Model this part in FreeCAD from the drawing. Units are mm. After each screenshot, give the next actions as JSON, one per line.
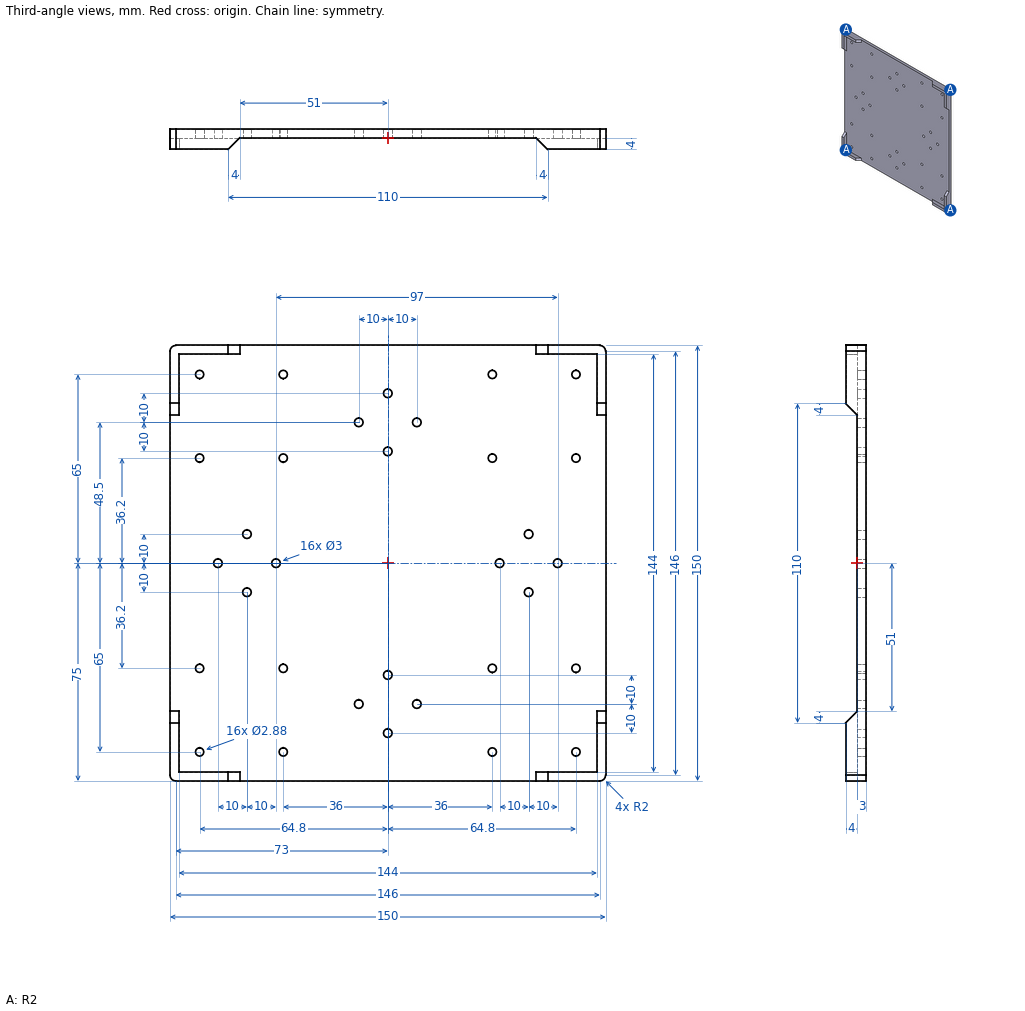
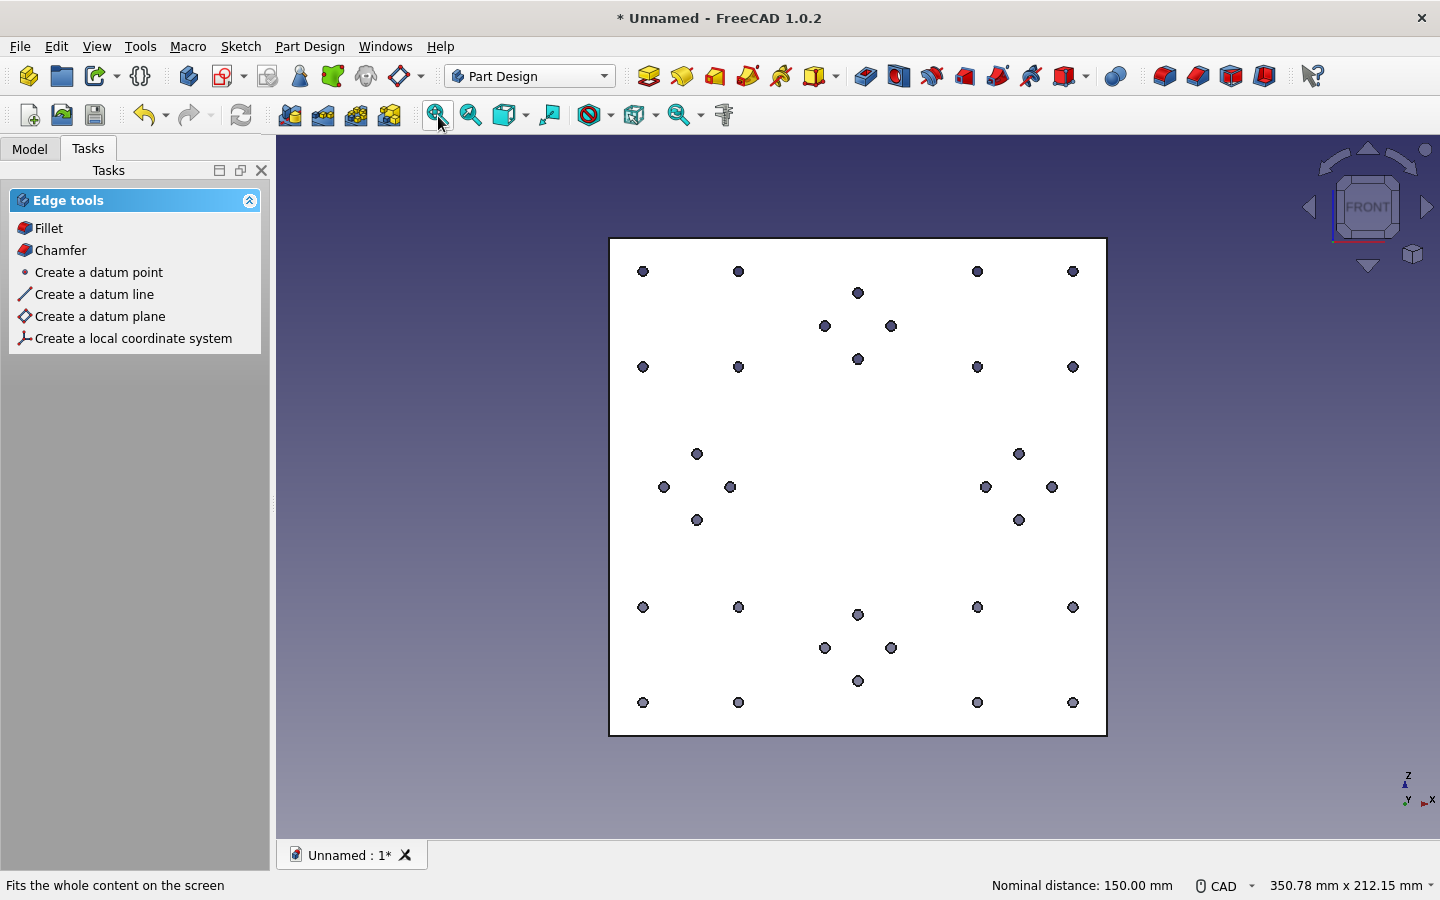
{"action": "key", "text": "3"}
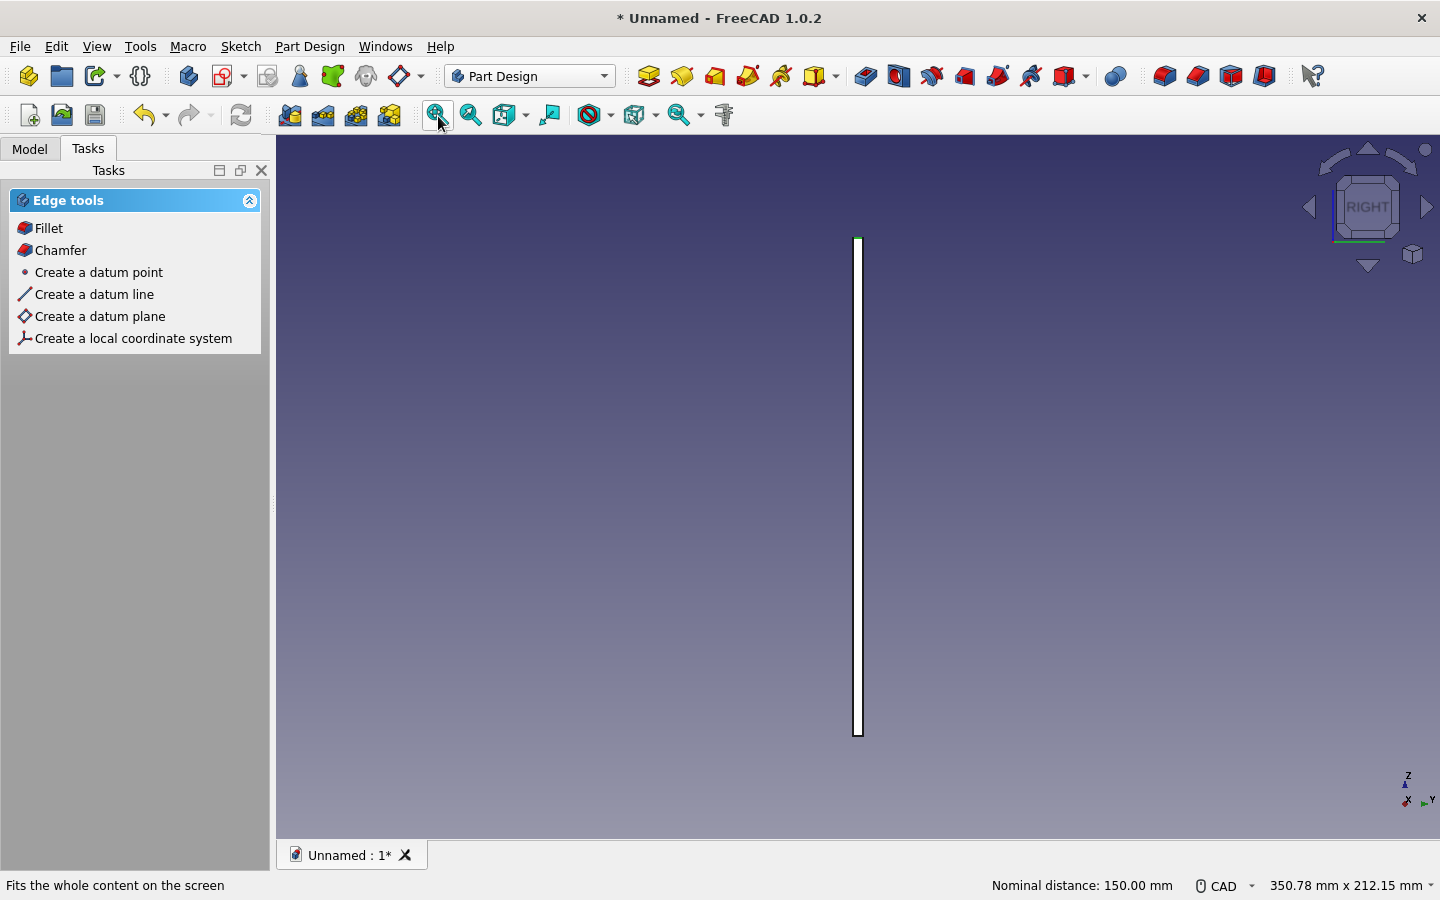
{"action": "scroll", "coordinate": [858, 735], "scroll_direction": "up", "scroll_amount": 7}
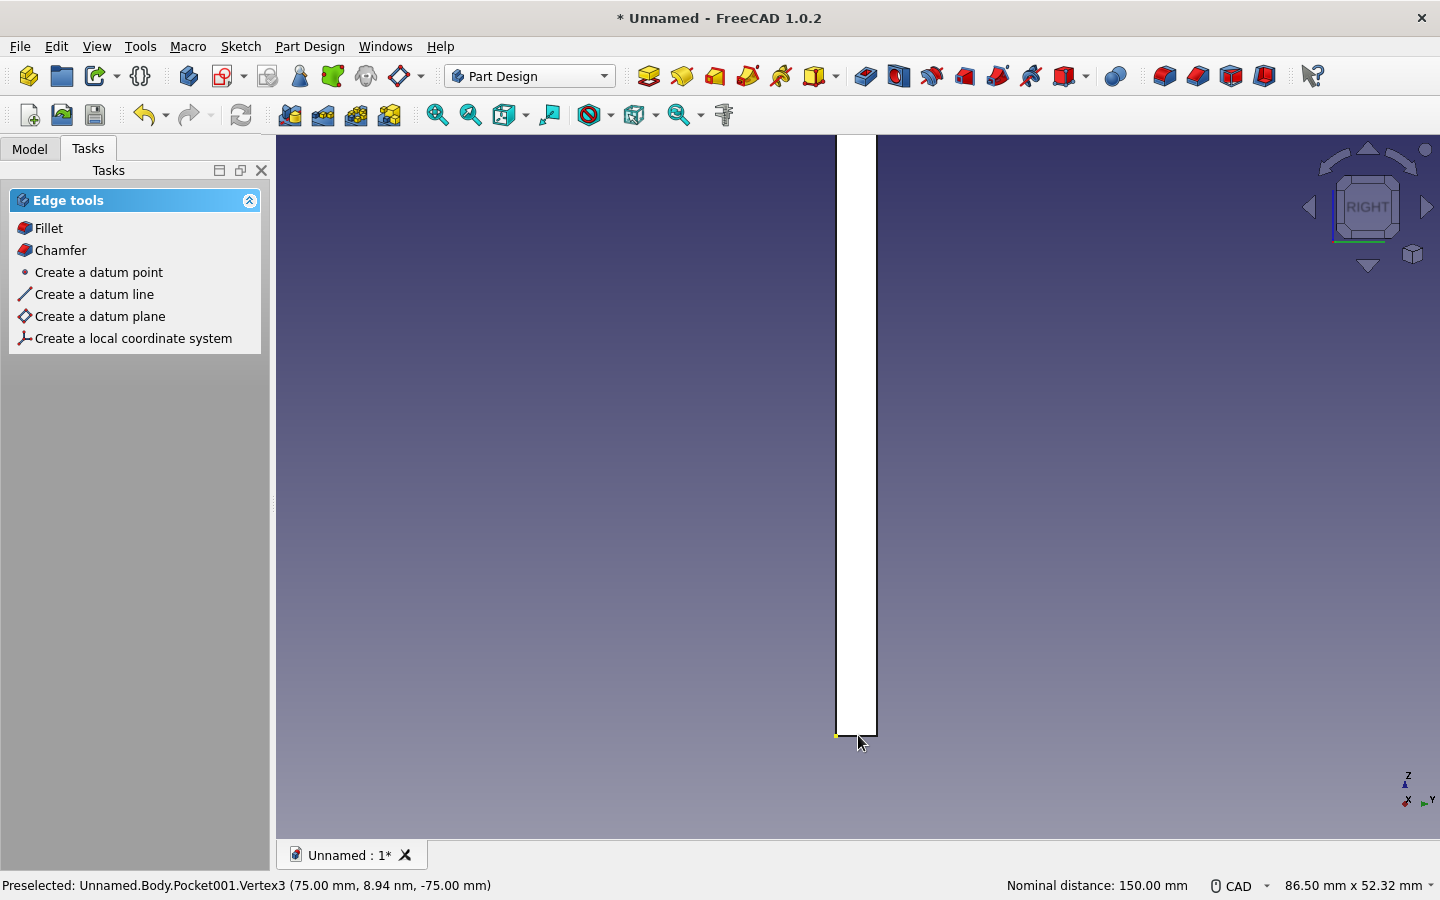
{"action": "left_click", "coordinate": [856, 735], "text": "ctrl"}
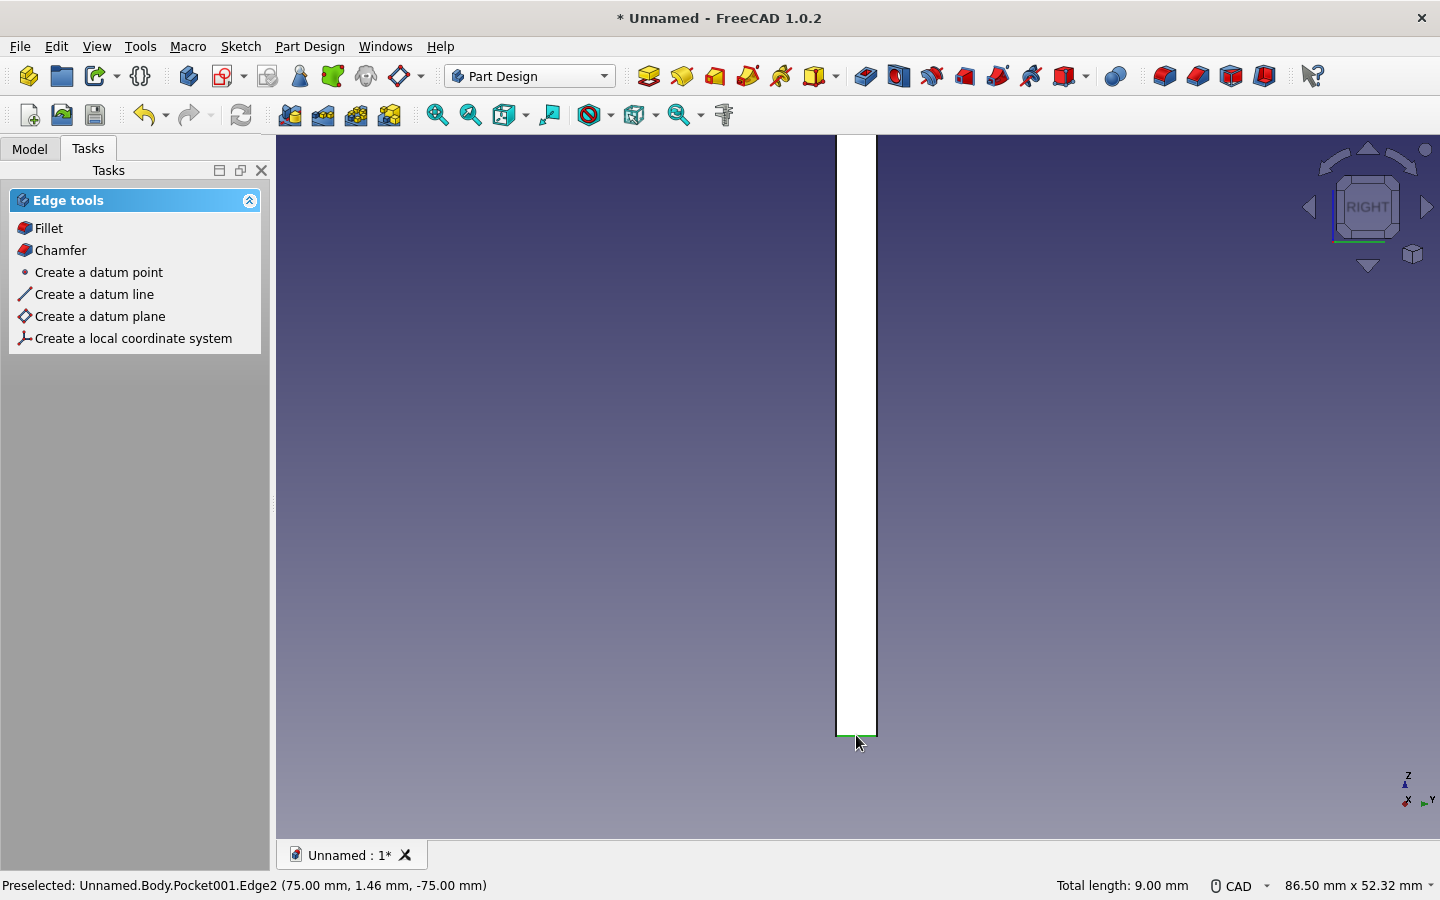
{"action": "key", "text": "v f"}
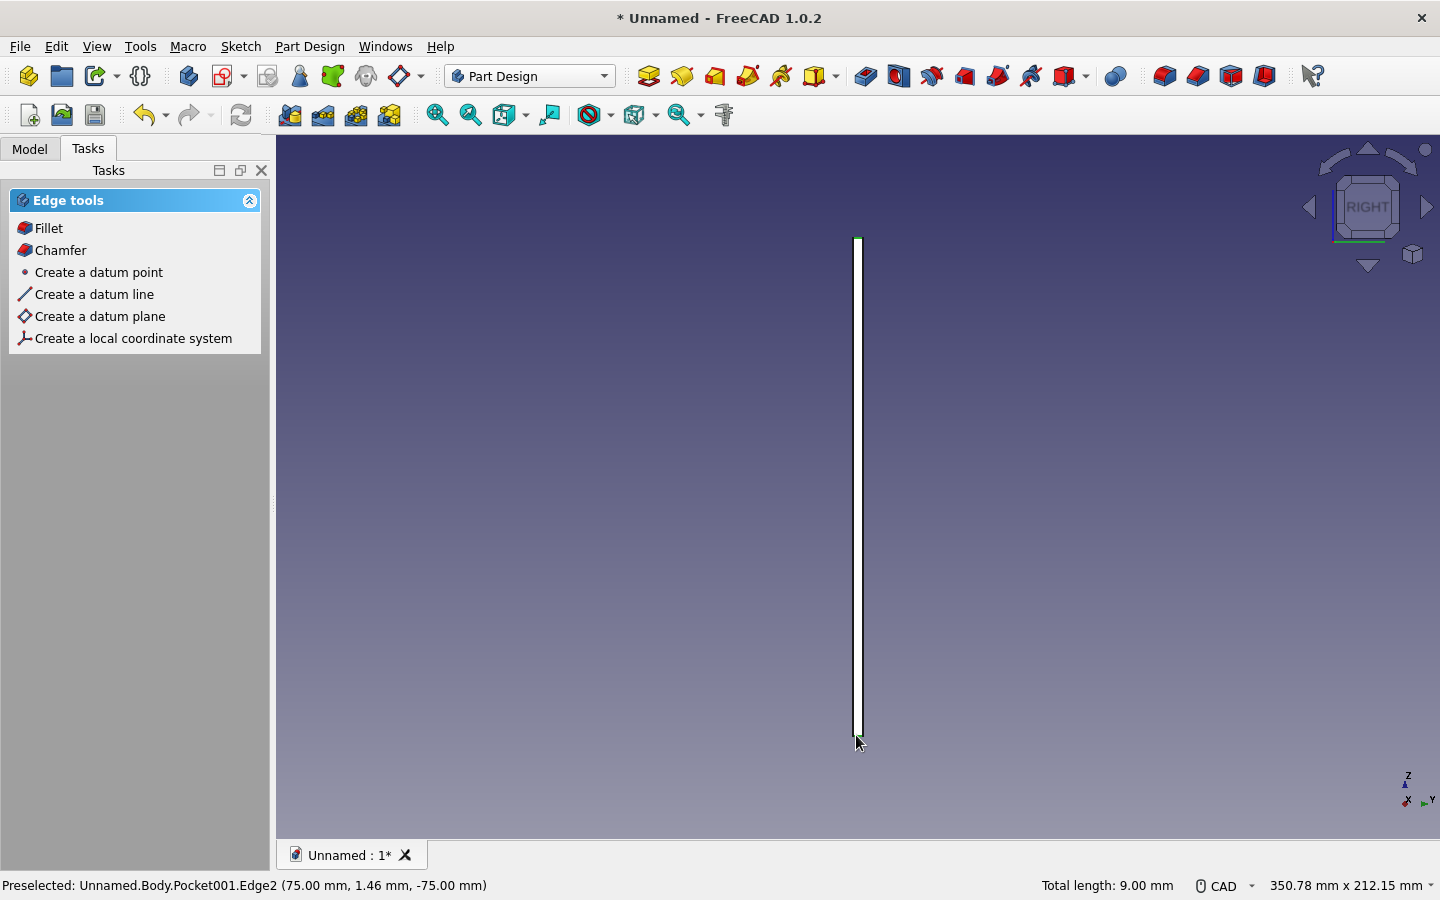
{"action": "key", "text": "5"}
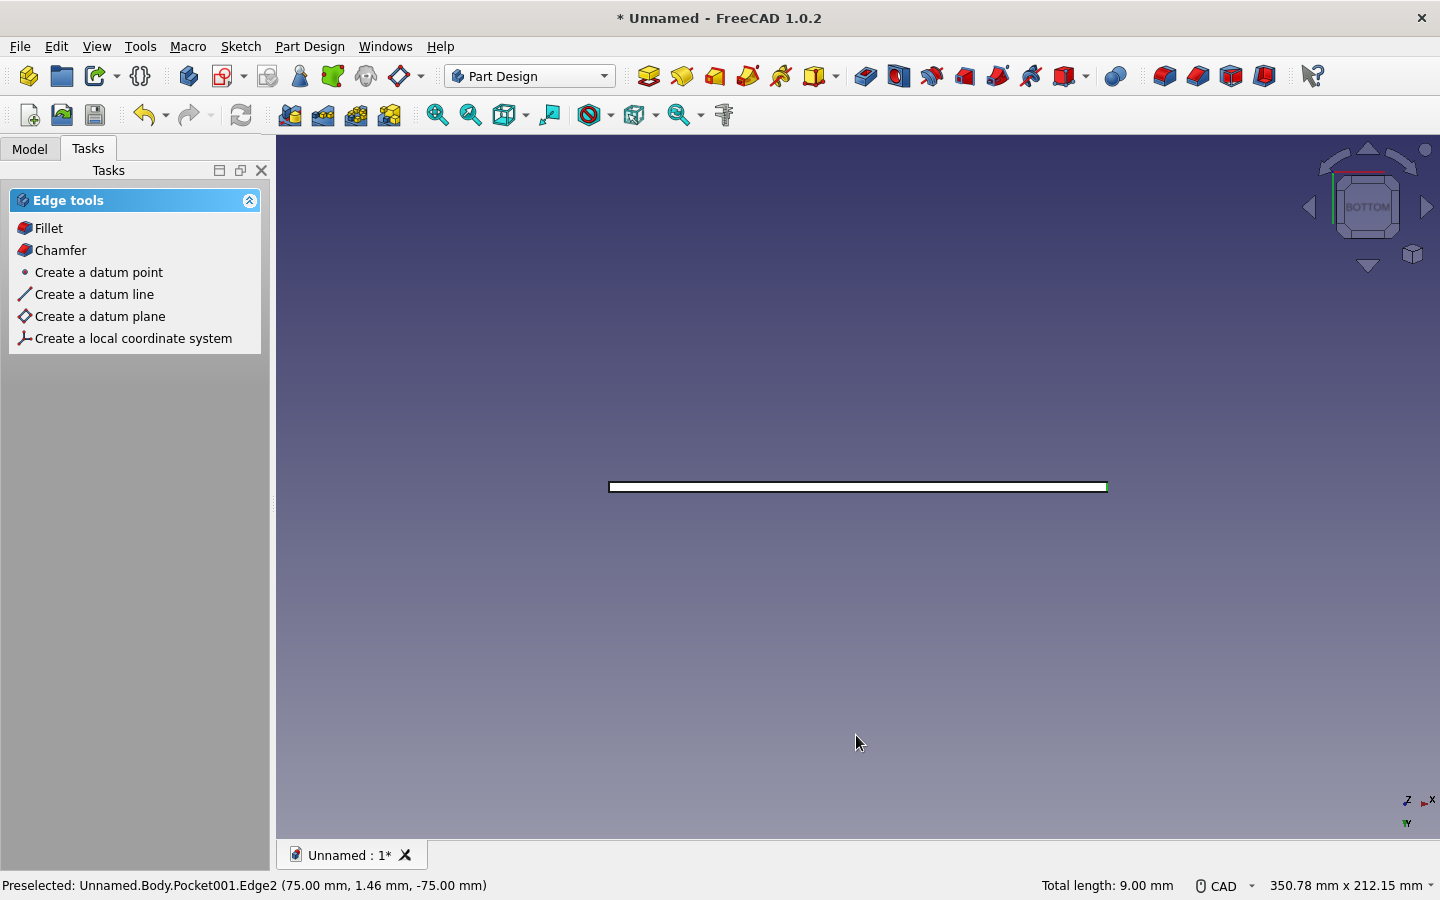
{"action": "key", "text": "v f"}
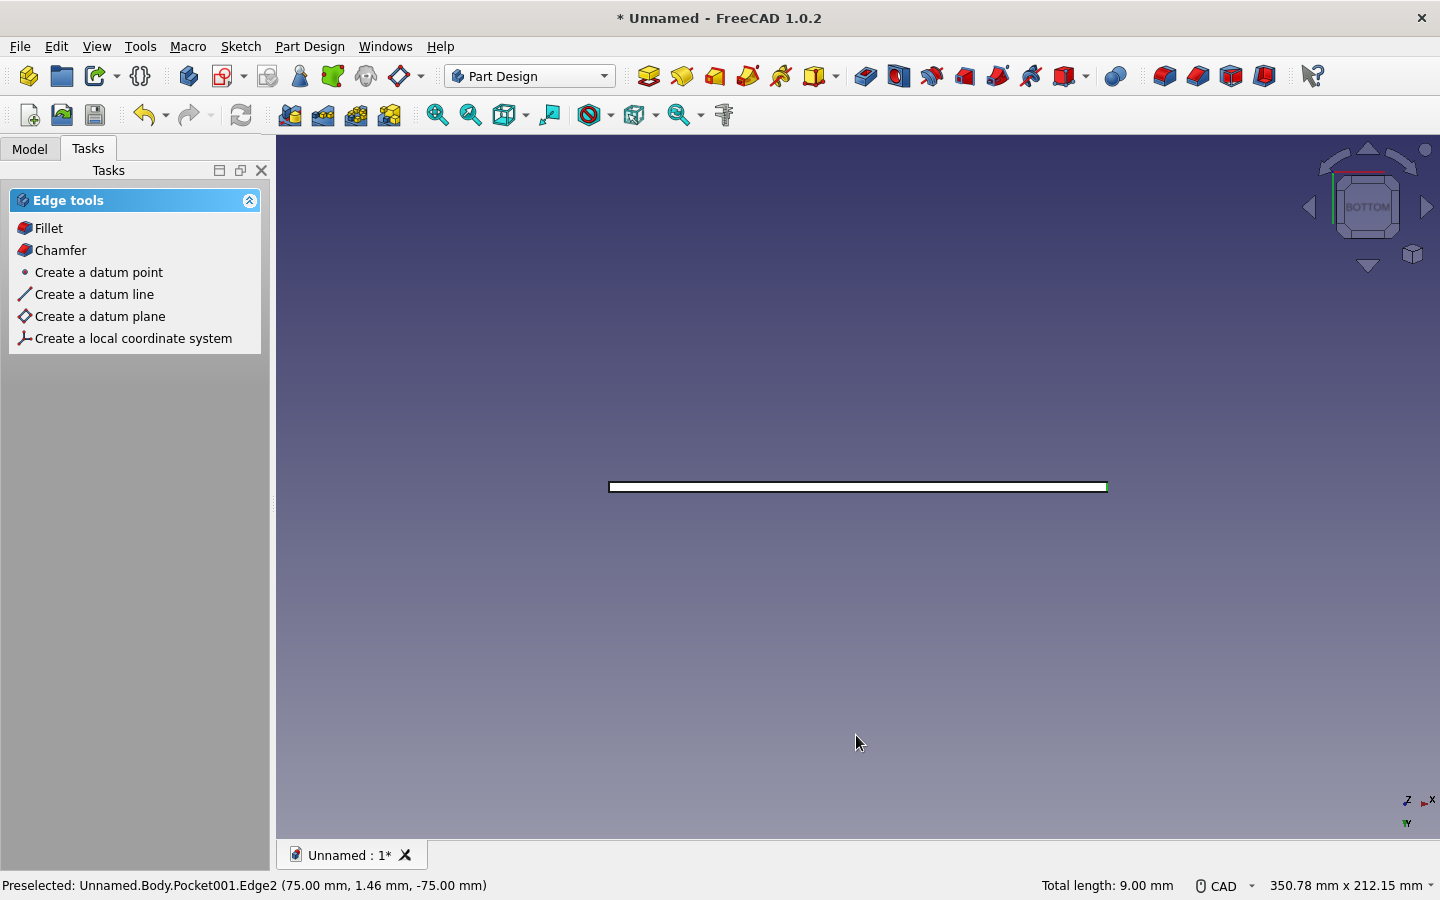
{"action": "left_click", "coordinate": [609, 488], "text": "ctrl"}